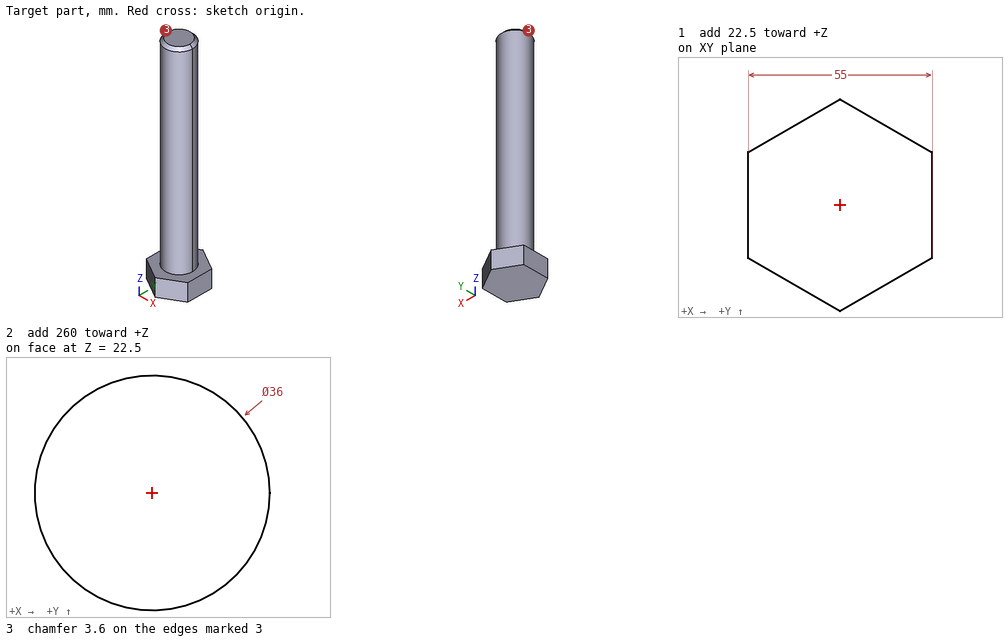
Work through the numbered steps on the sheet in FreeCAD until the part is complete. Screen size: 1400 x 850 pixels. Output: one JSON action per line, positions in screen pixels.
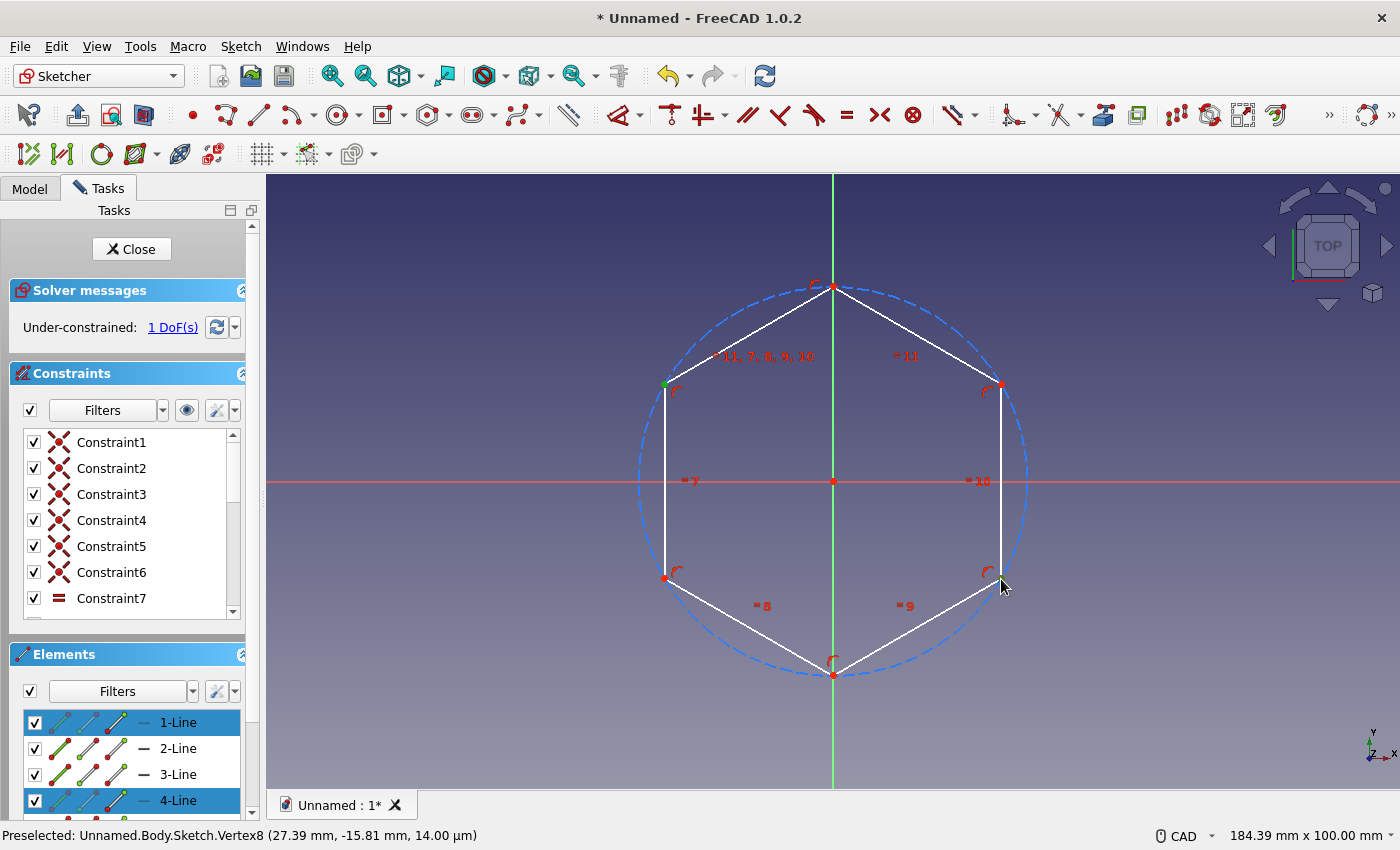
{"action": "key", "text": "l"}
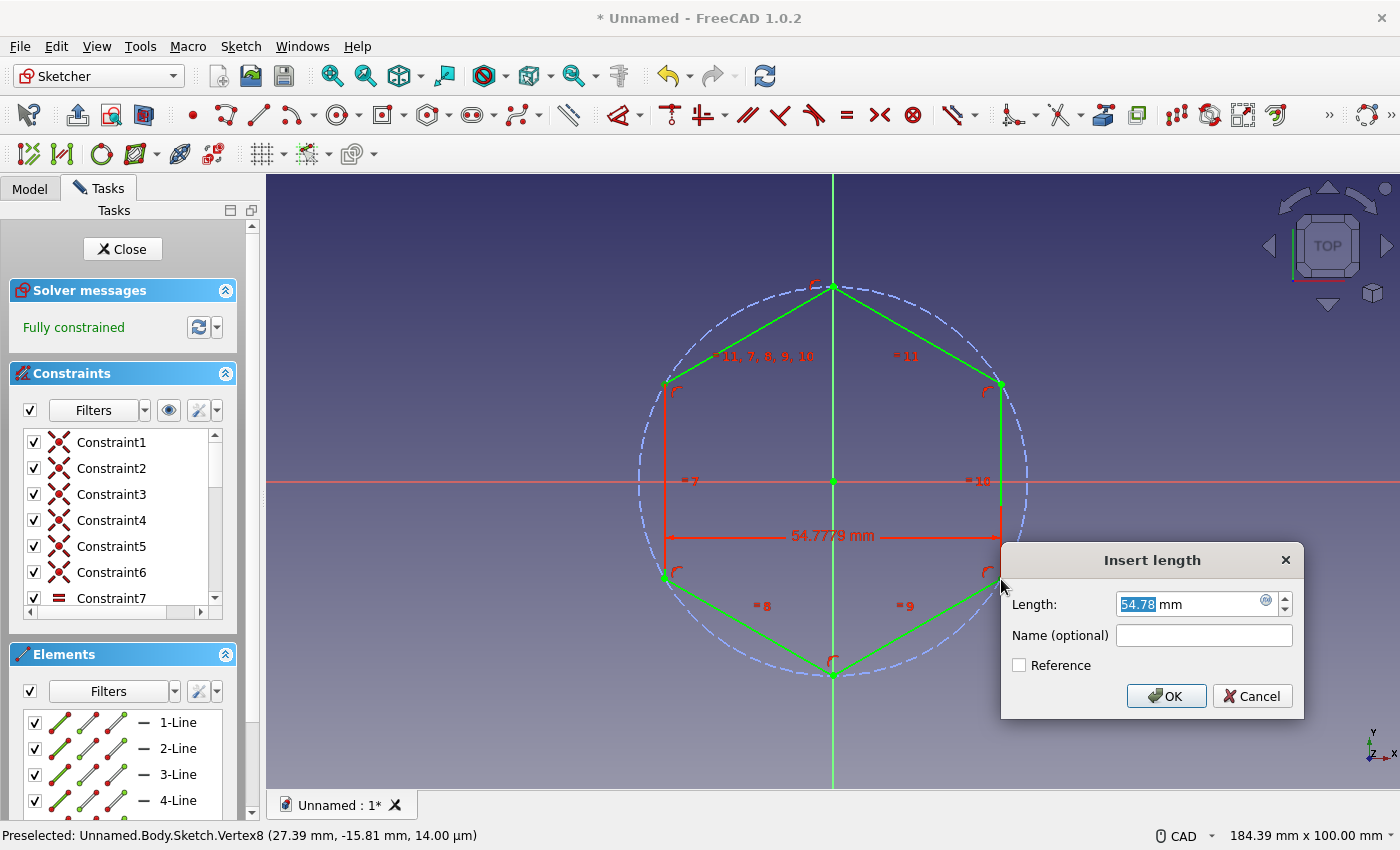
{"action": "type", "text": "55"}
{"action": "key", "text": "Return"}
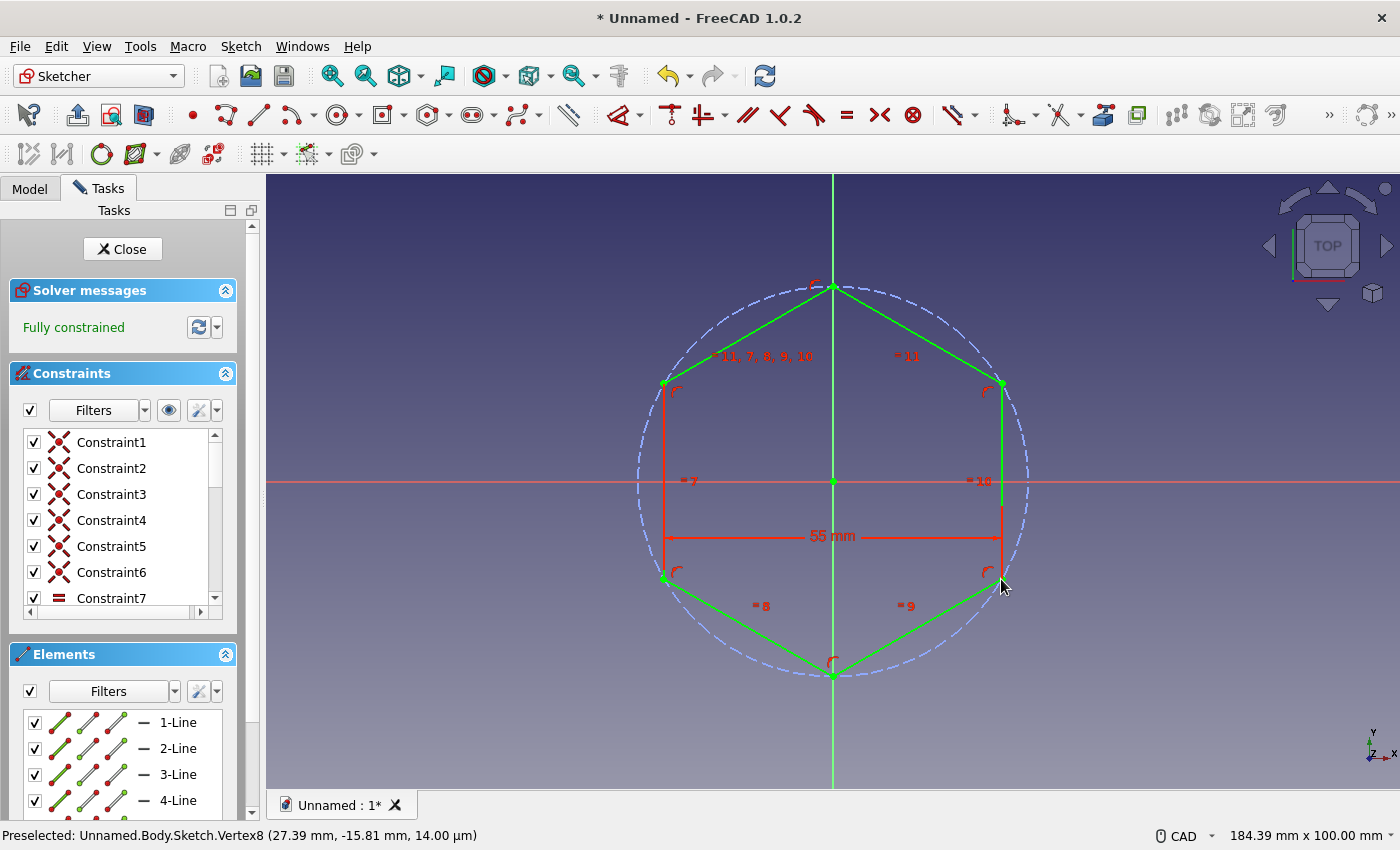
{"action": "left_click", "coordinate": [123, 249]}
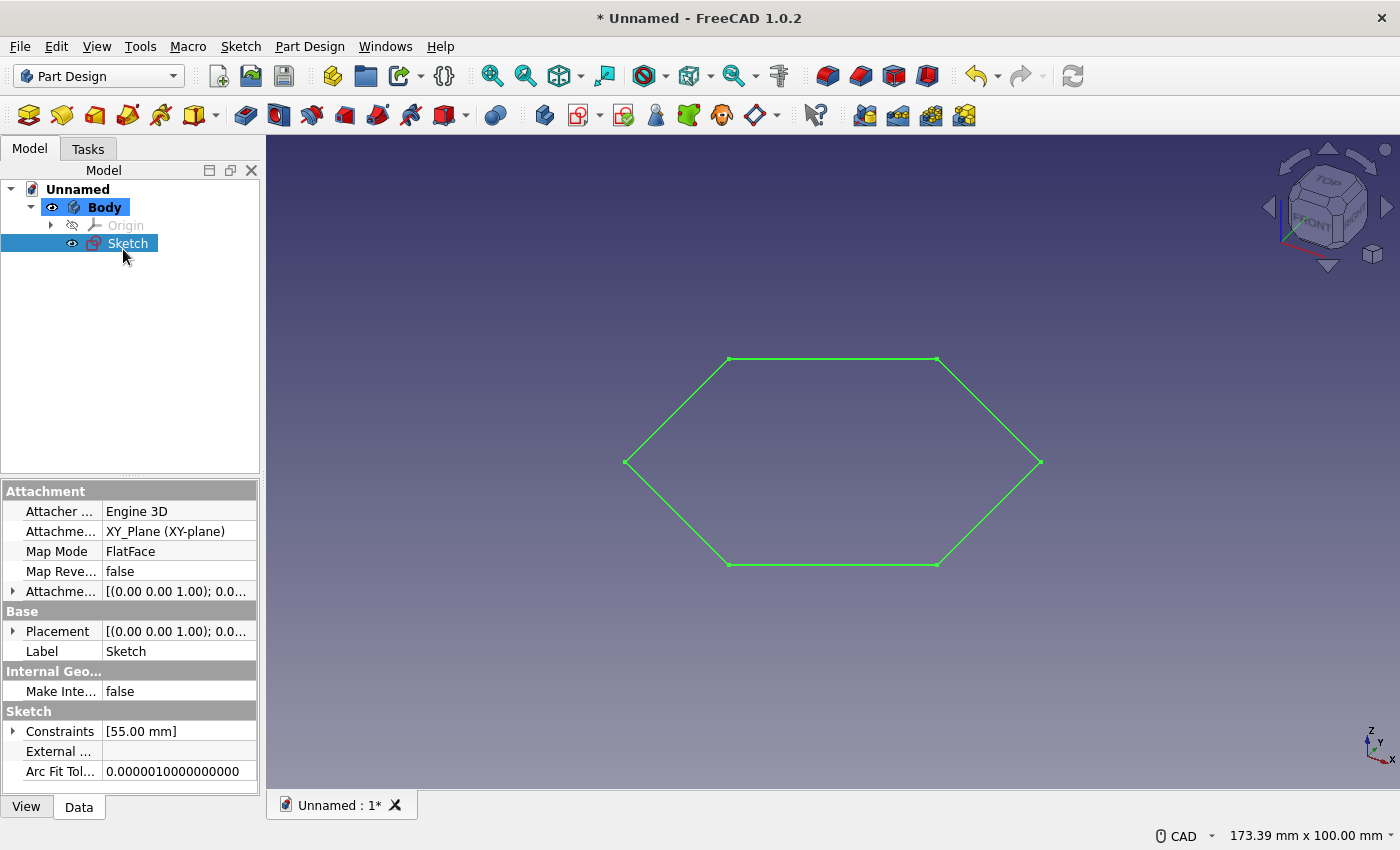
{"action": "left_click", "coordinate": [29, 116]}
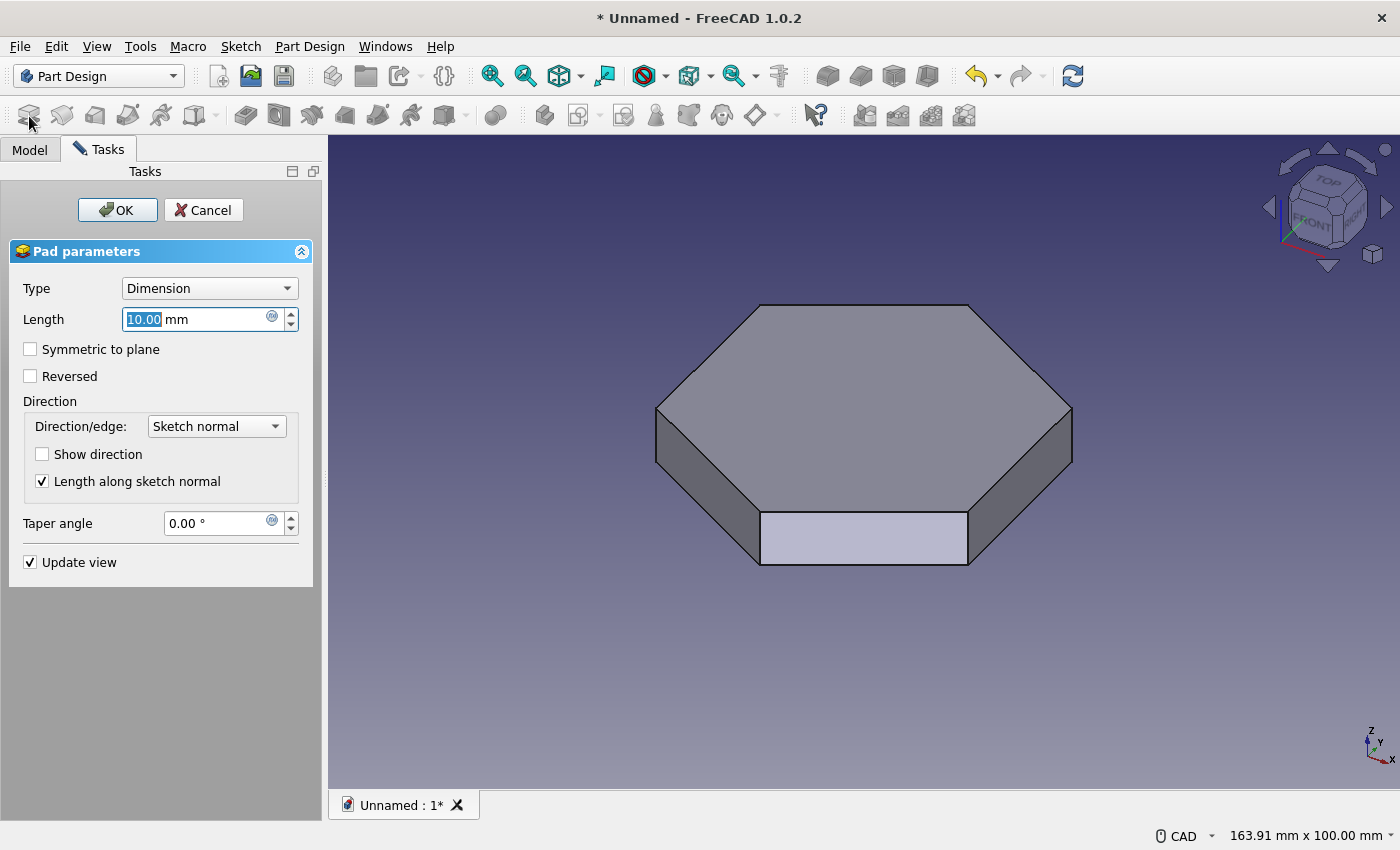
{"action": "type", "text": "22.5"}
{"action": "key", "text": "Tab"}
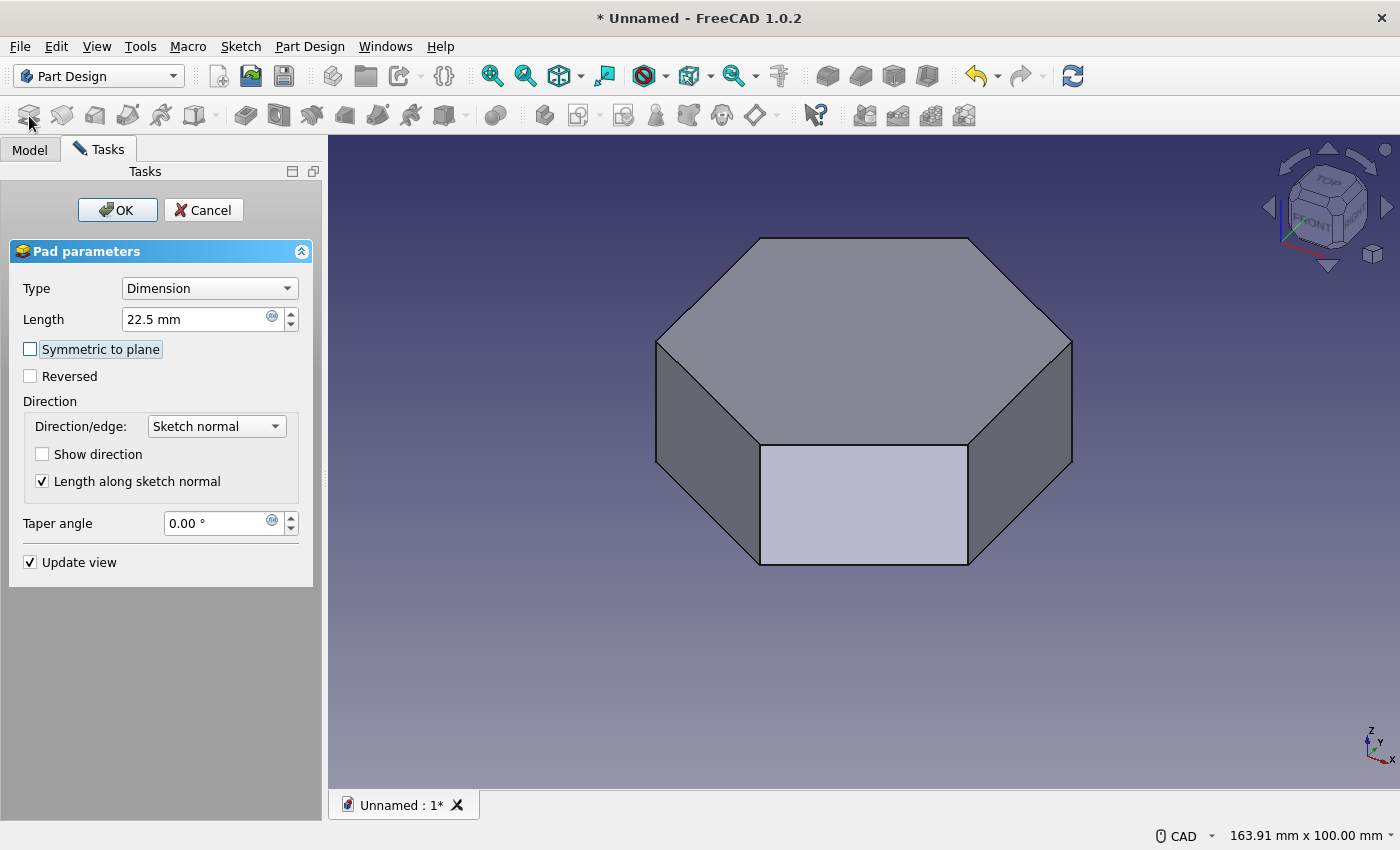
{"action": "left_click", "coordinate": [118, 210]}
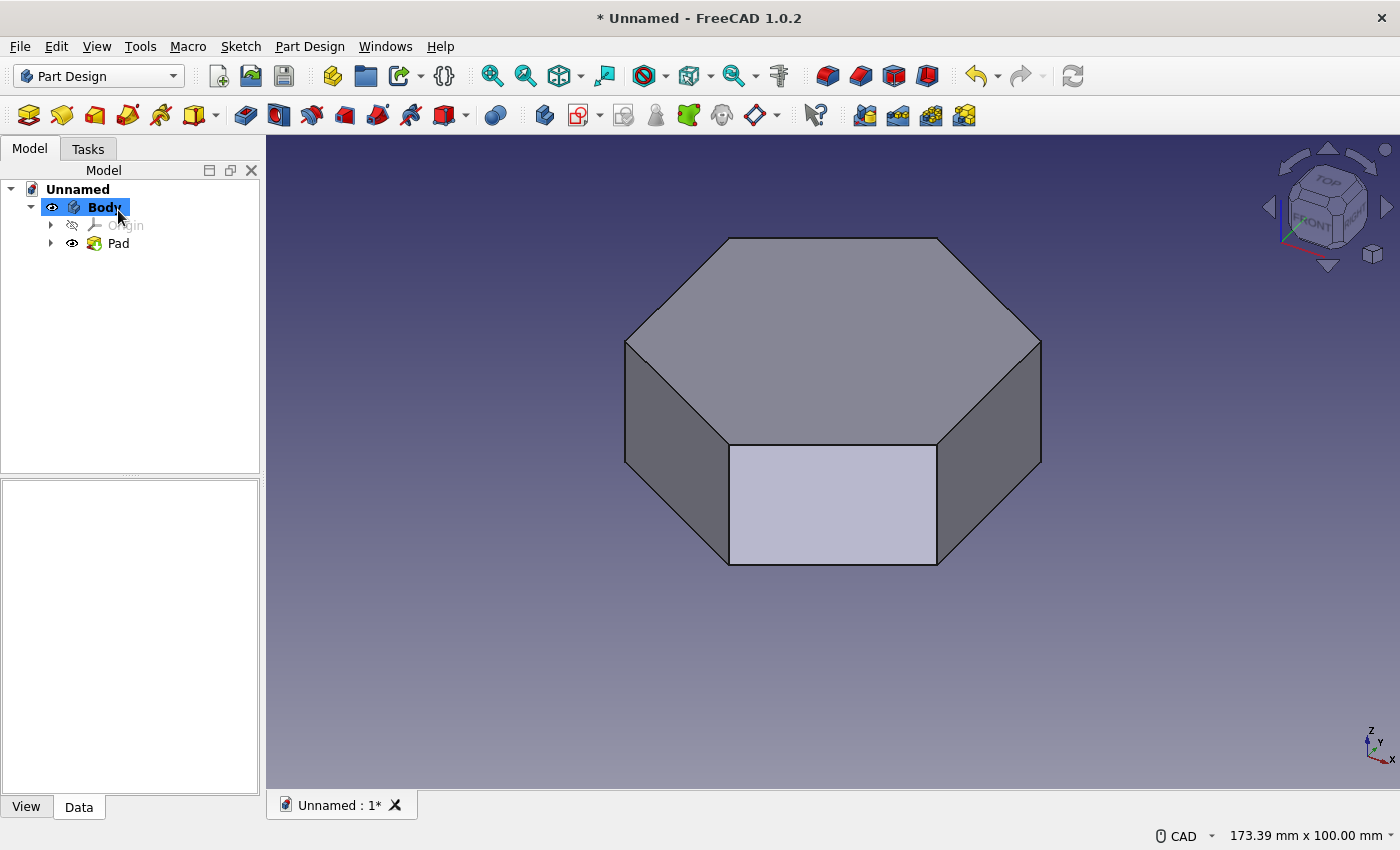
{"action": "left_click", "coordinate": [833, 340]}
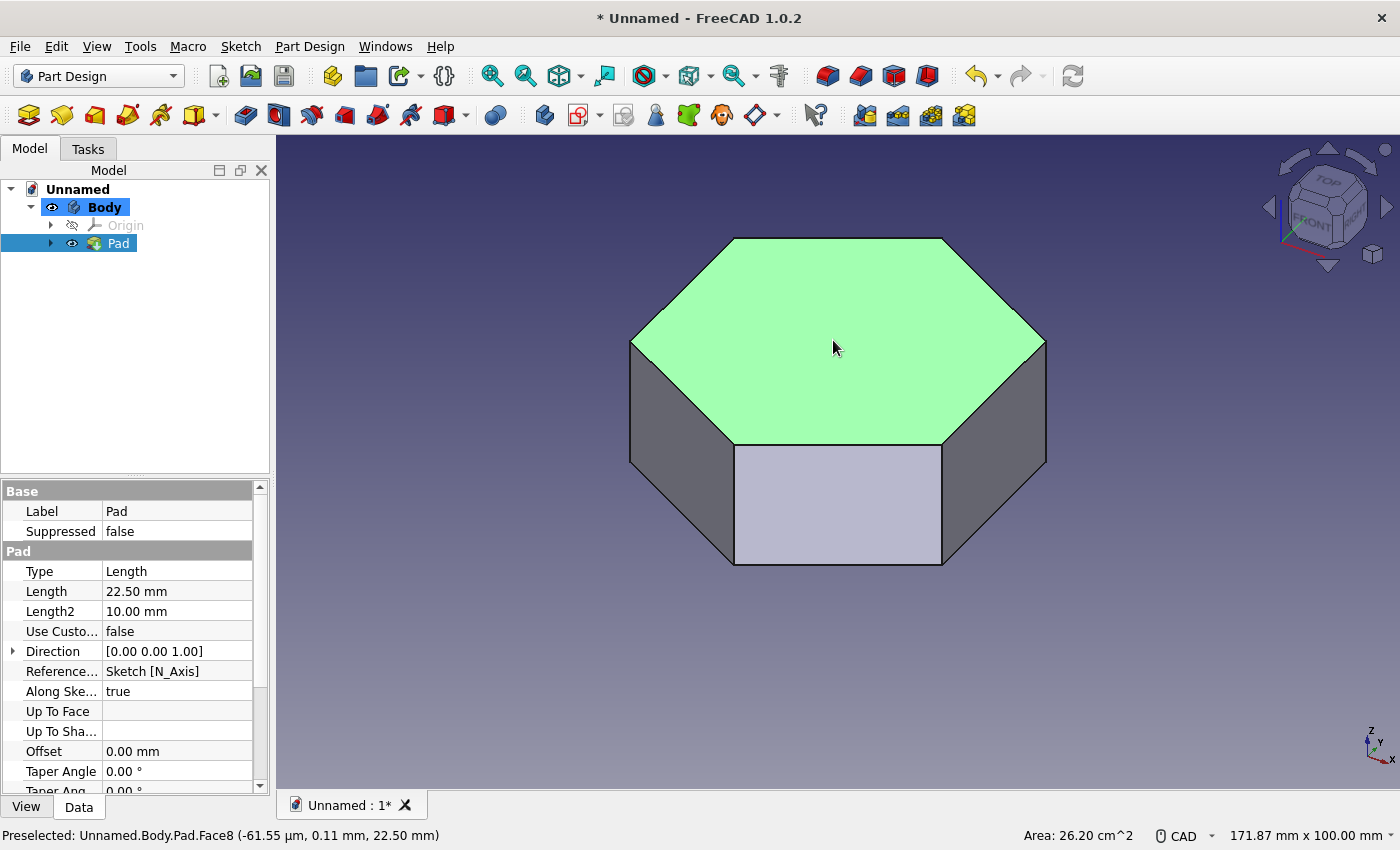
{"action": "left_click", "coordinate": [578, 116]}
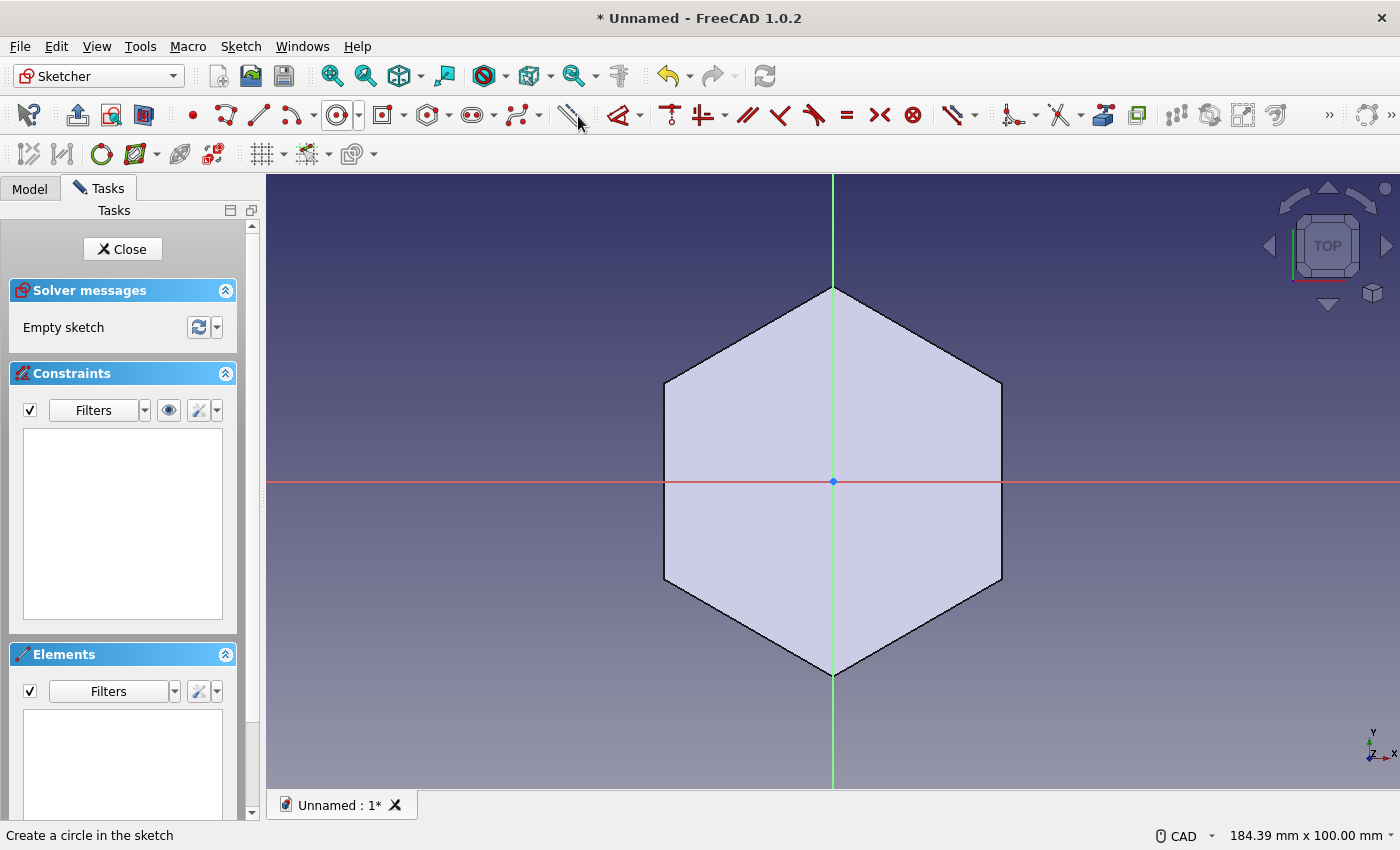
{"action": "scroll", "coordinate": [916, 481], "scroll_direction": "up", "scroll_amount": 3}